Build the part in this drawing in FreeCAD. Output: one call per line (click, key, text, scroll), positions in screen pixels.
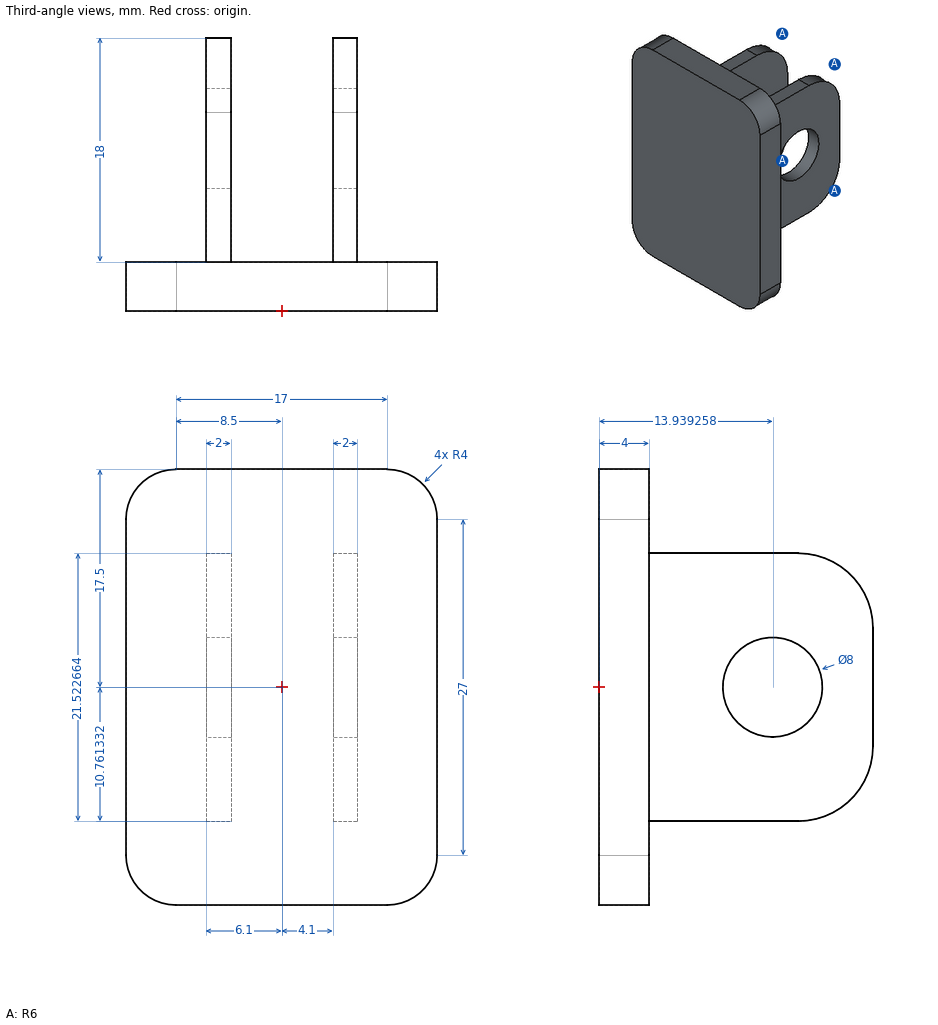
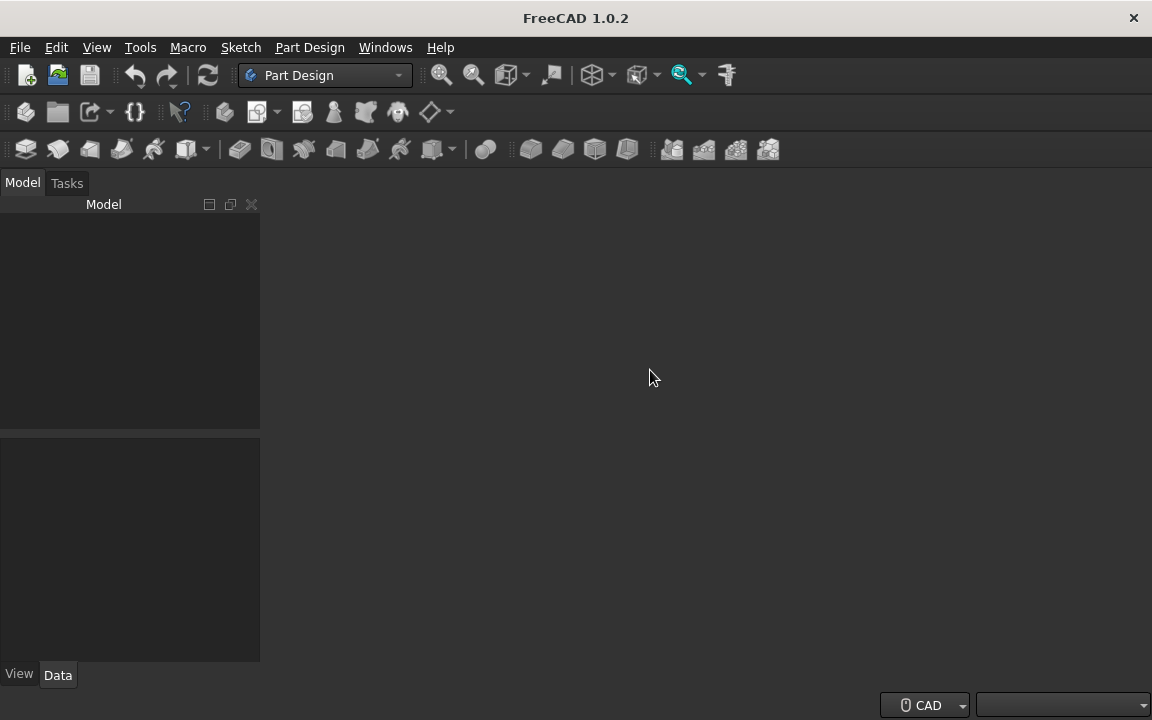
click(26, 76)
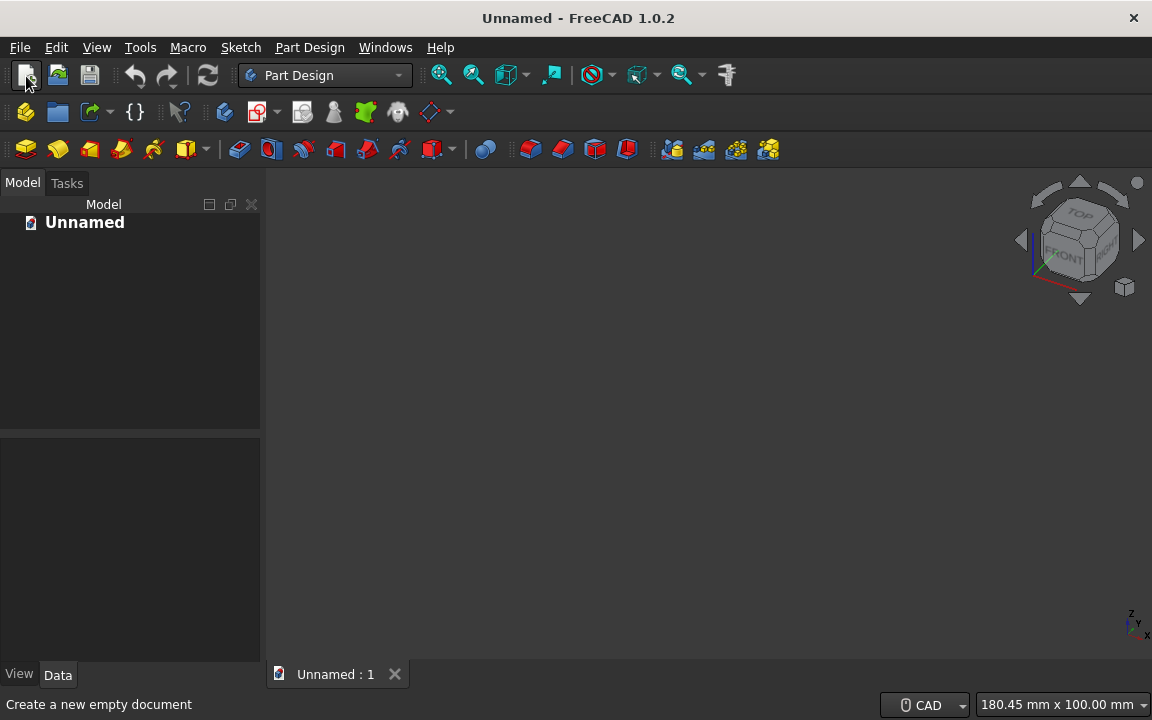
click(258, 112)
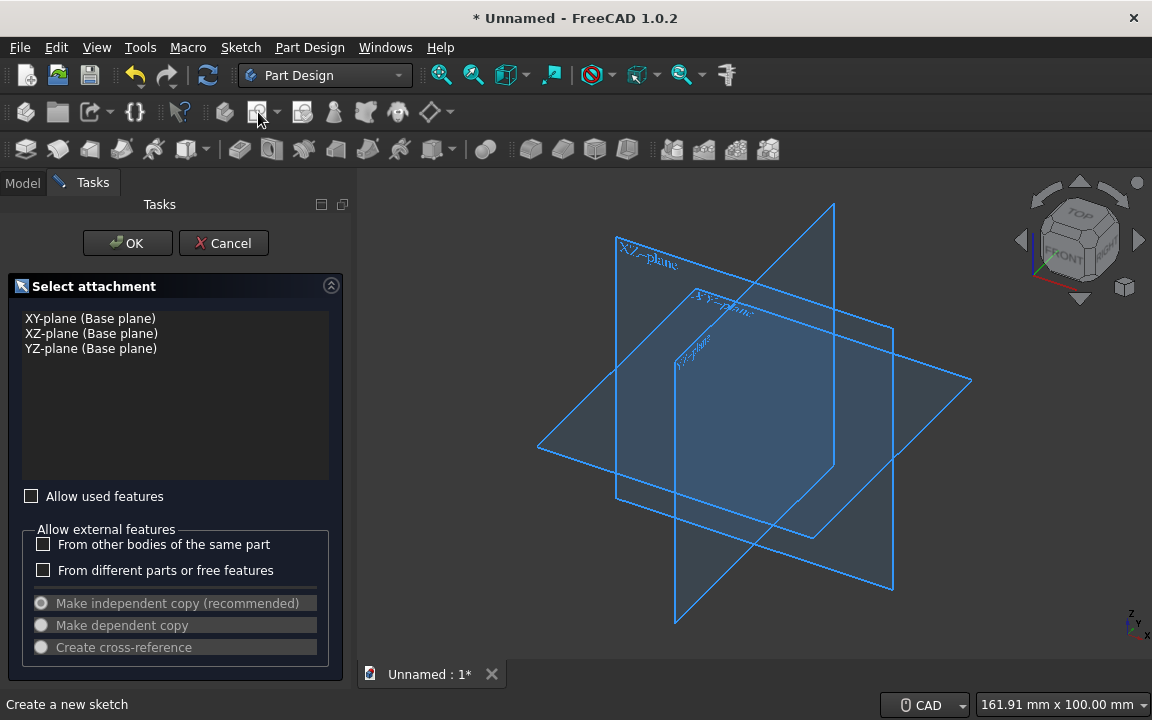
click(82, 334)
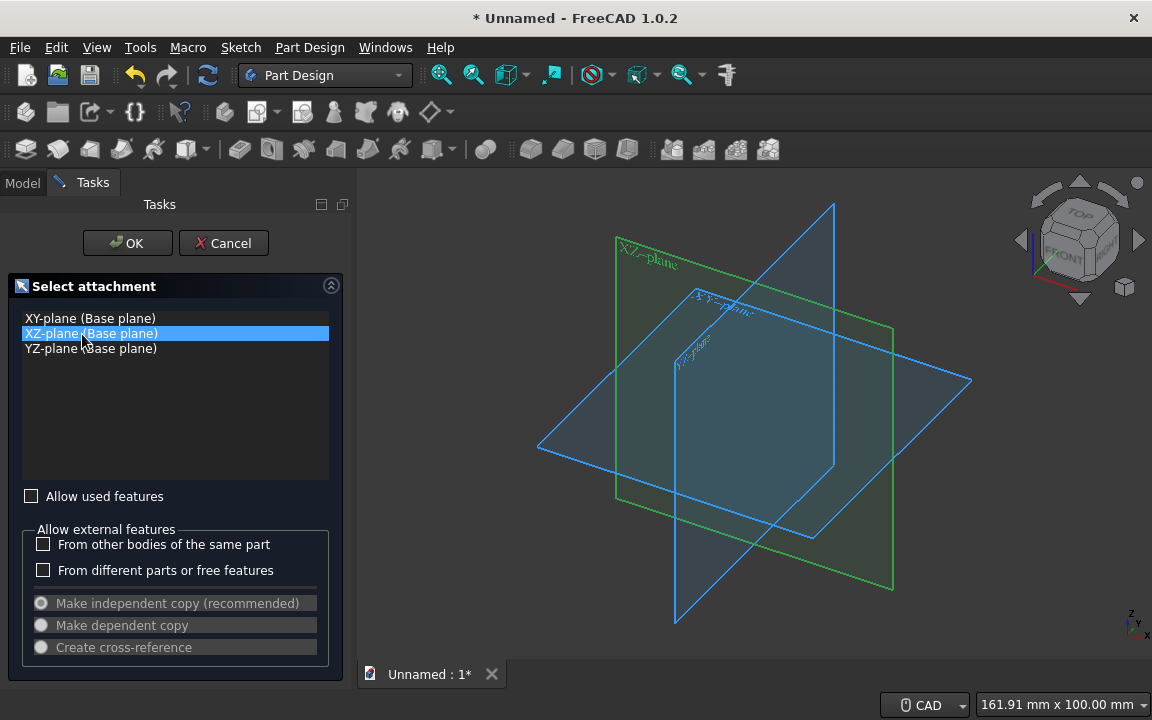
click(128, 243)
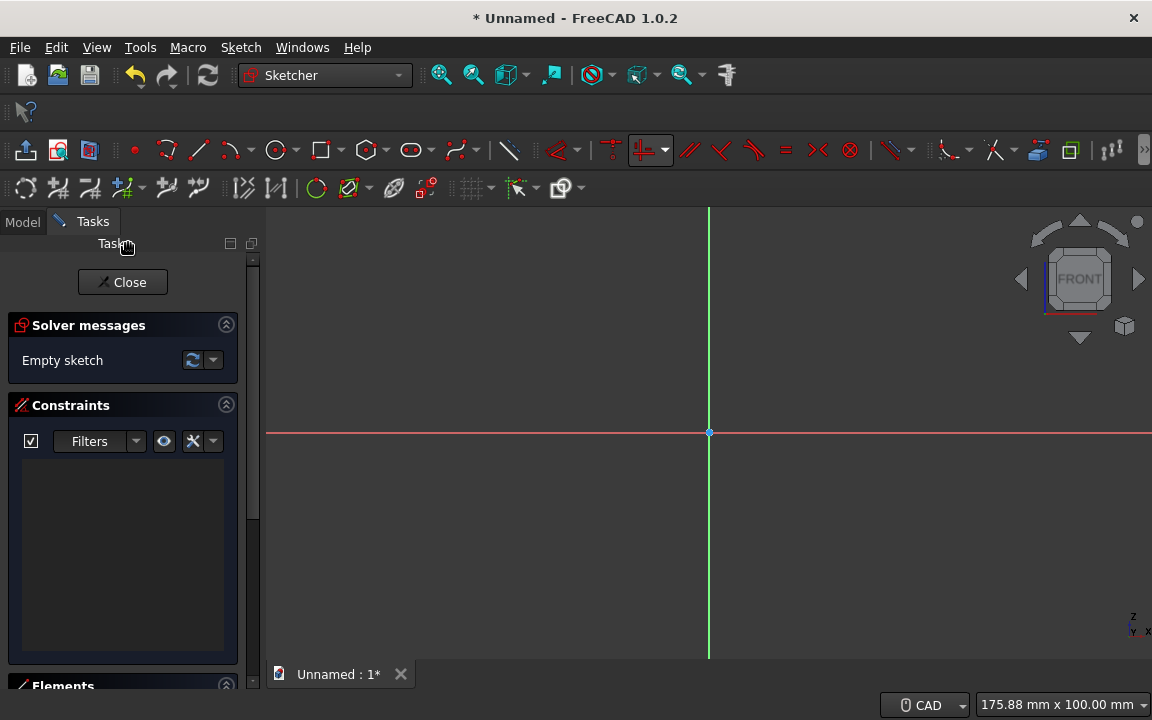
scroll(792, 433, up, 3)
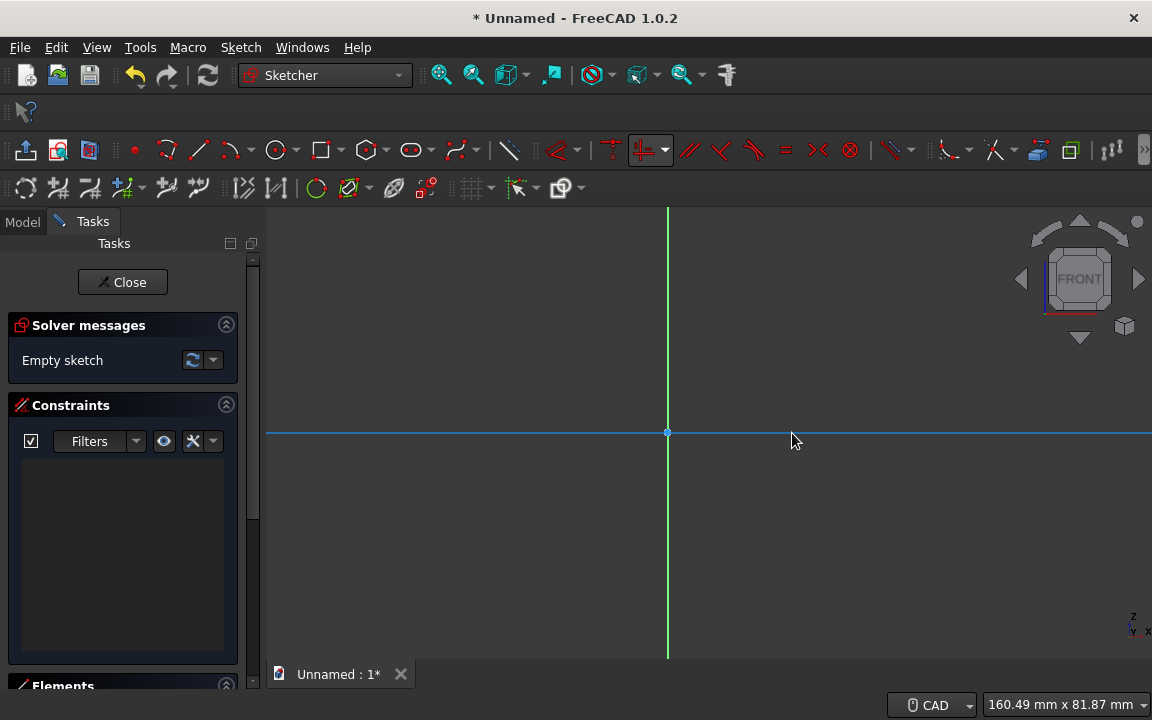
click(200, 150)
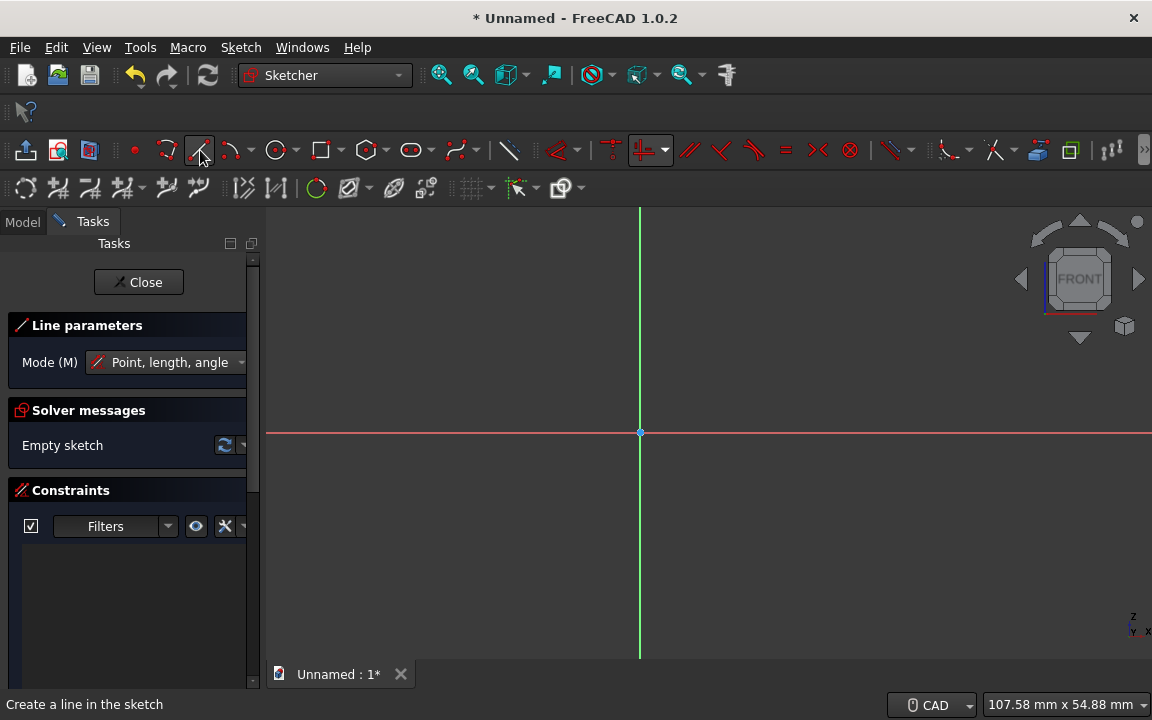
click(570, 288)
click(710, 288)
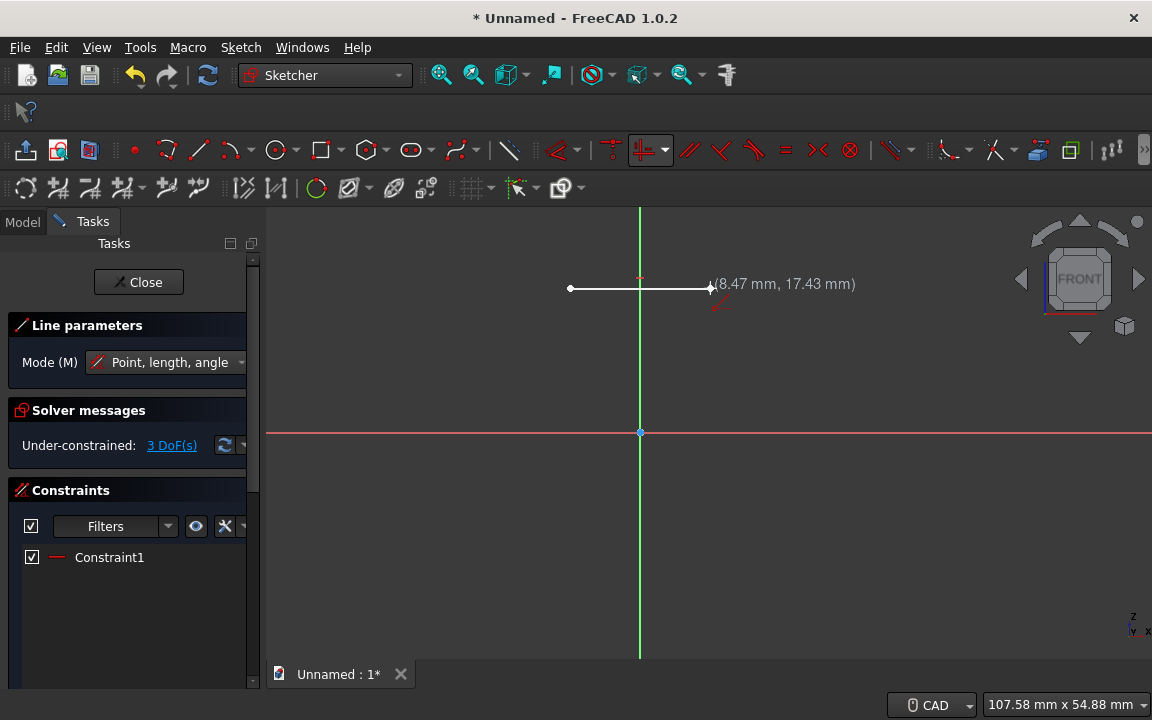
click(743, 321)
click(743, 544)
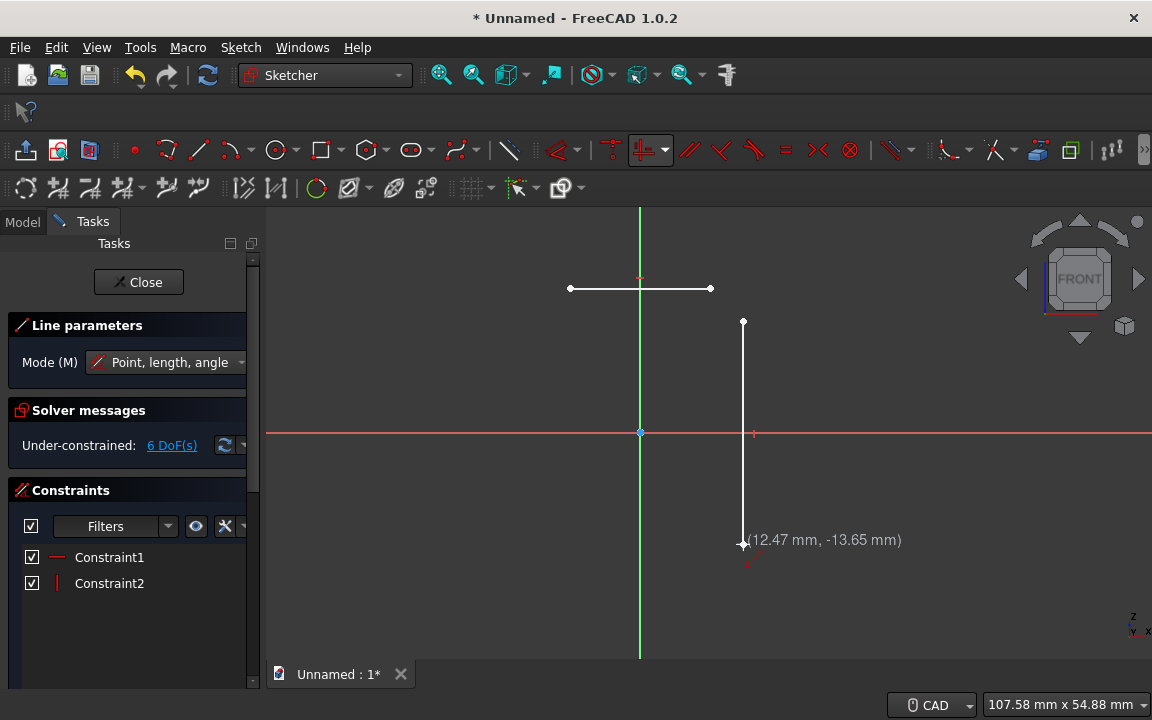
click(710, 577)
click(570, 577)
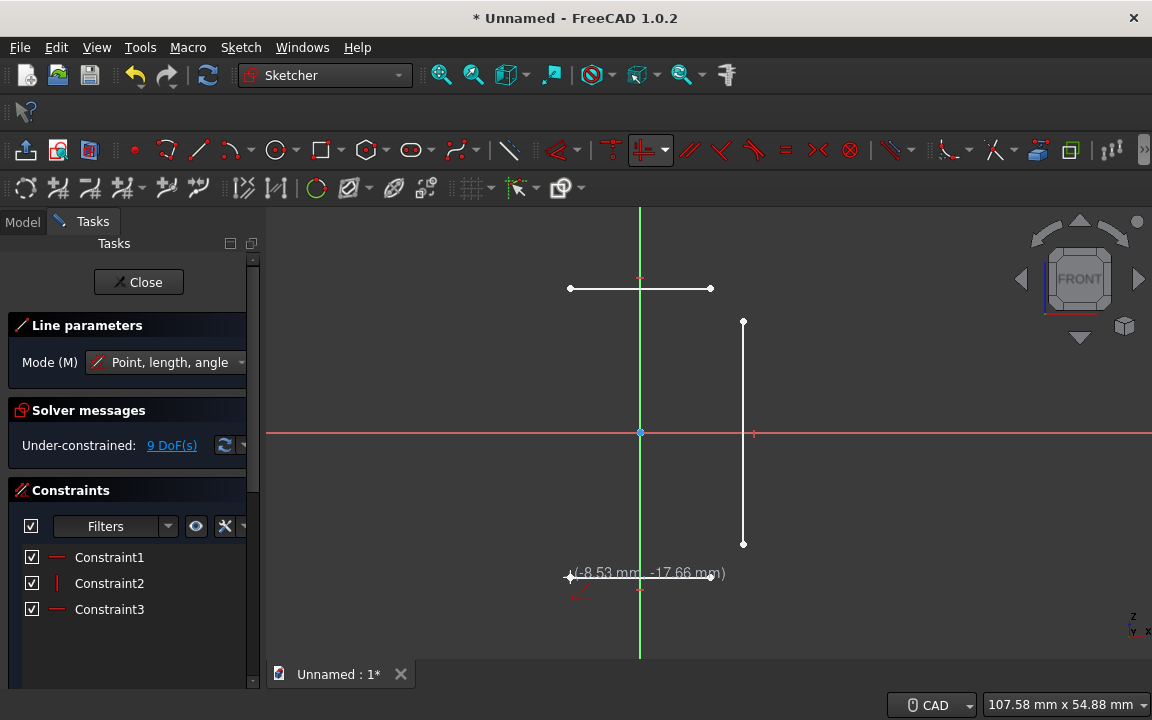
click(537, 544)
click(537, 321)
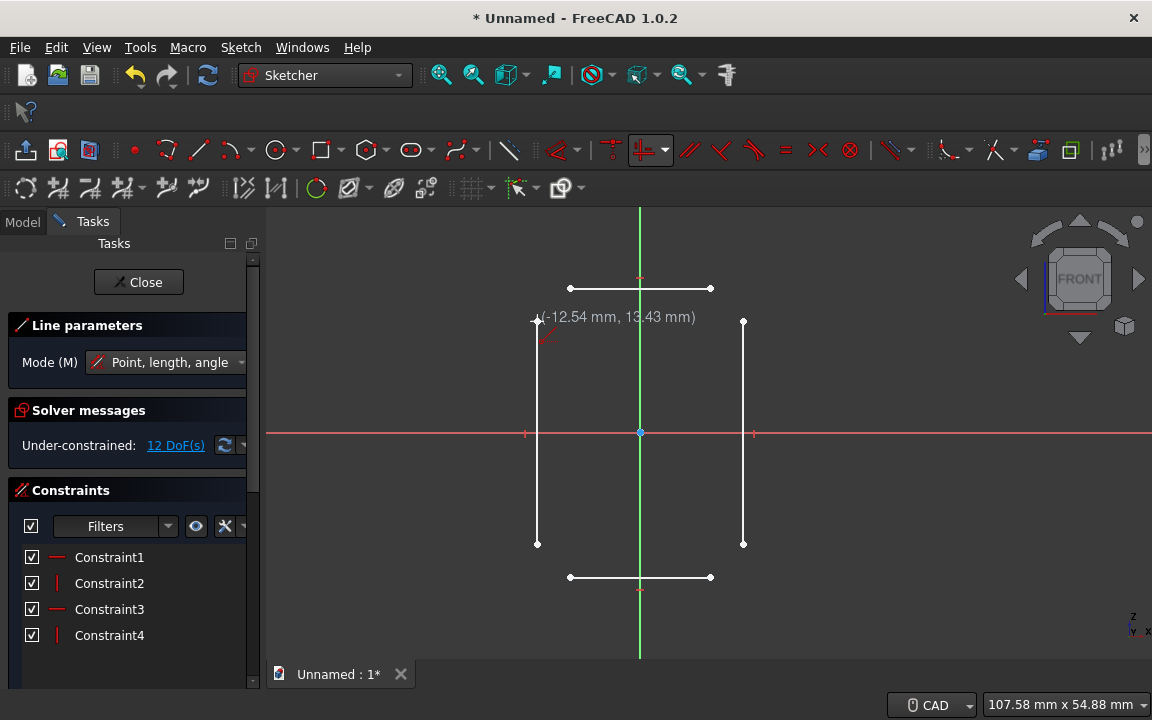
key(g)
key(3)
key(a)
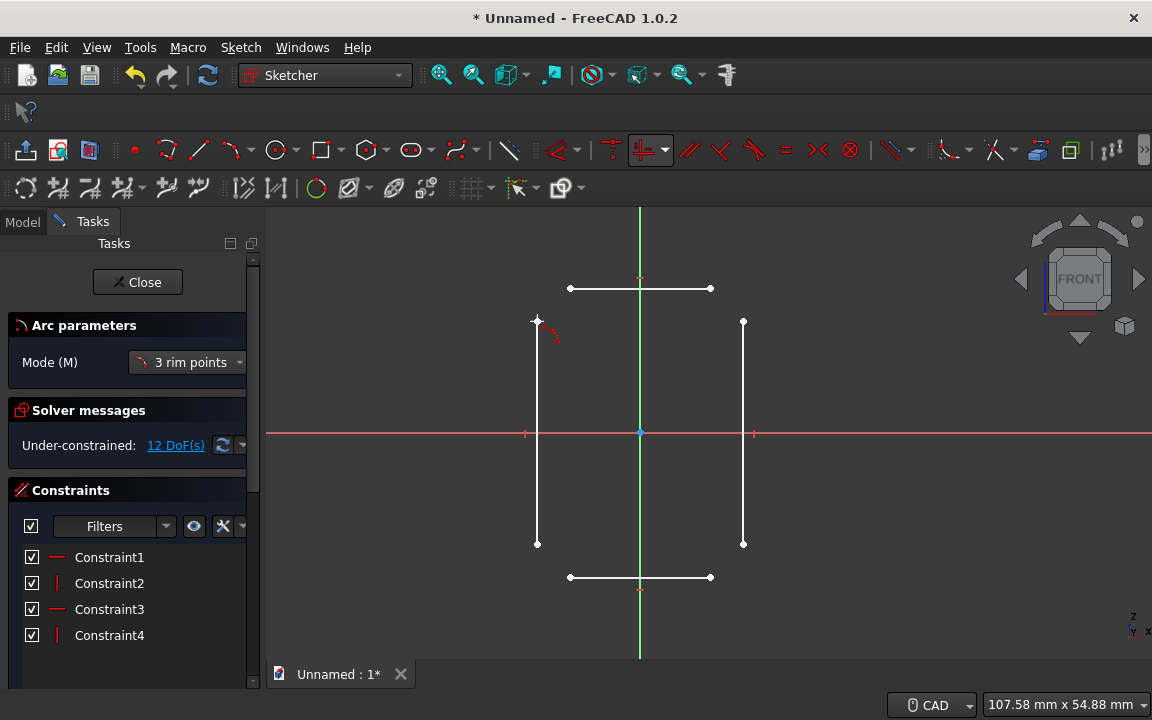
click(710, 289)
click(743, 322)